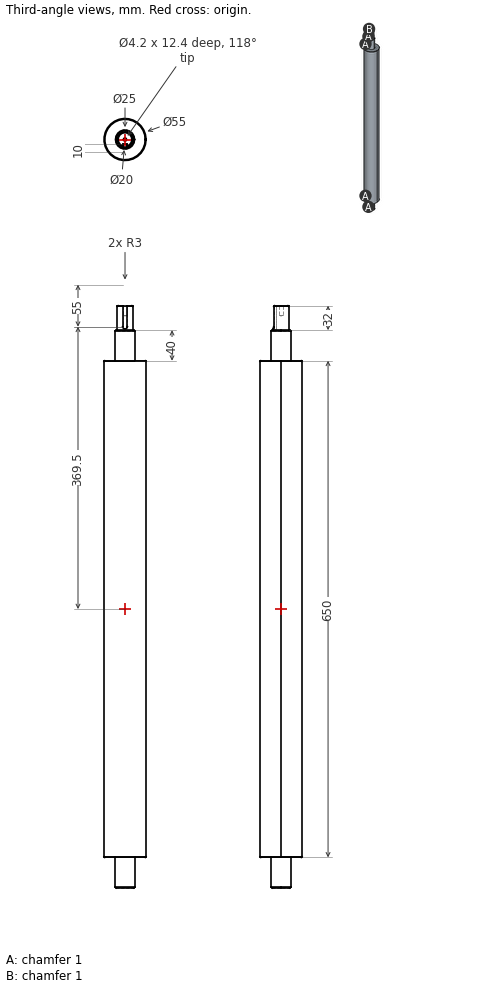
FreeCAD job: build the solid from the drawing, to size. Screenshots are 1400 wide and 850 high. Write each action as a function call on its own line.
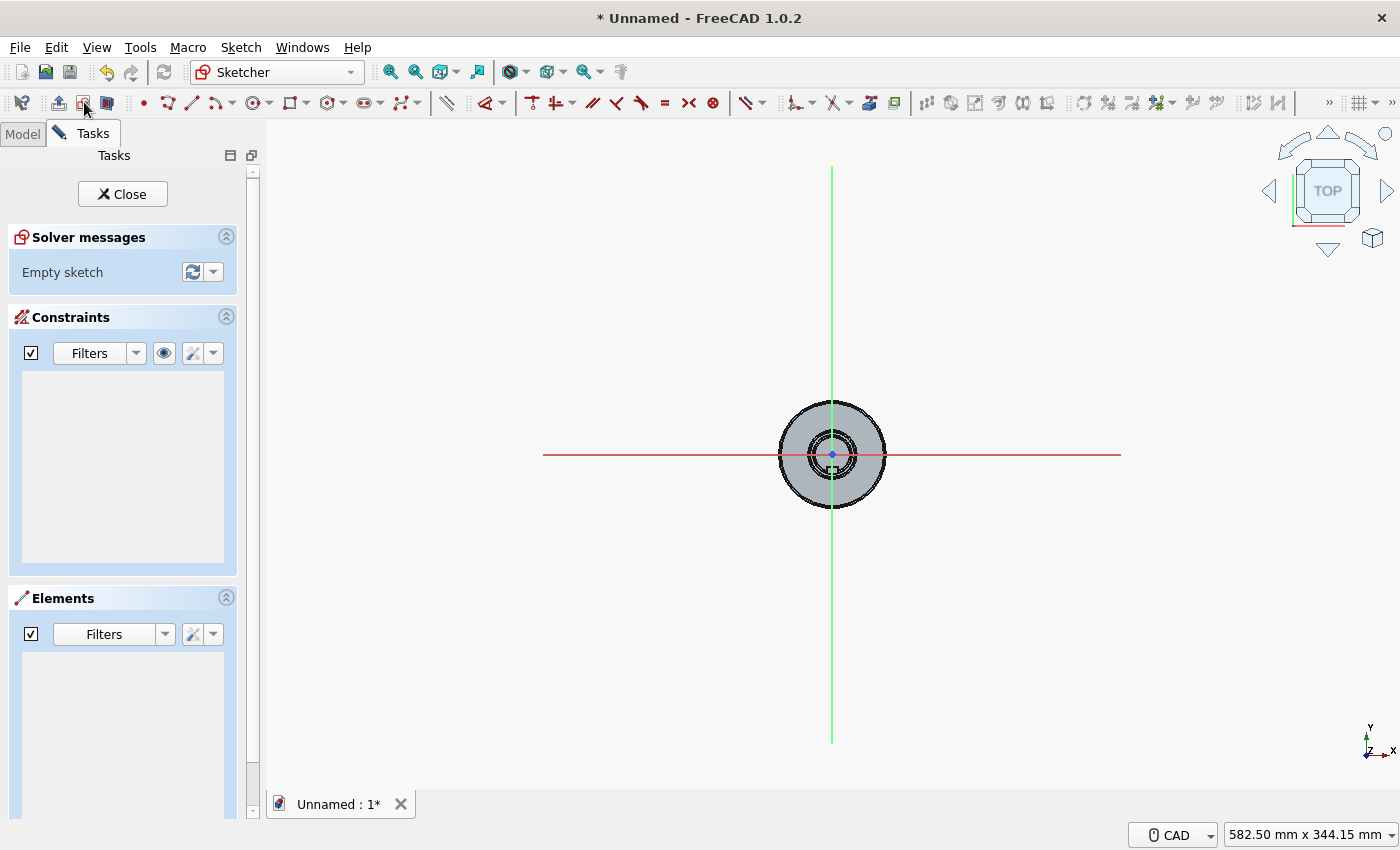
scroll(836, 455, up, 15)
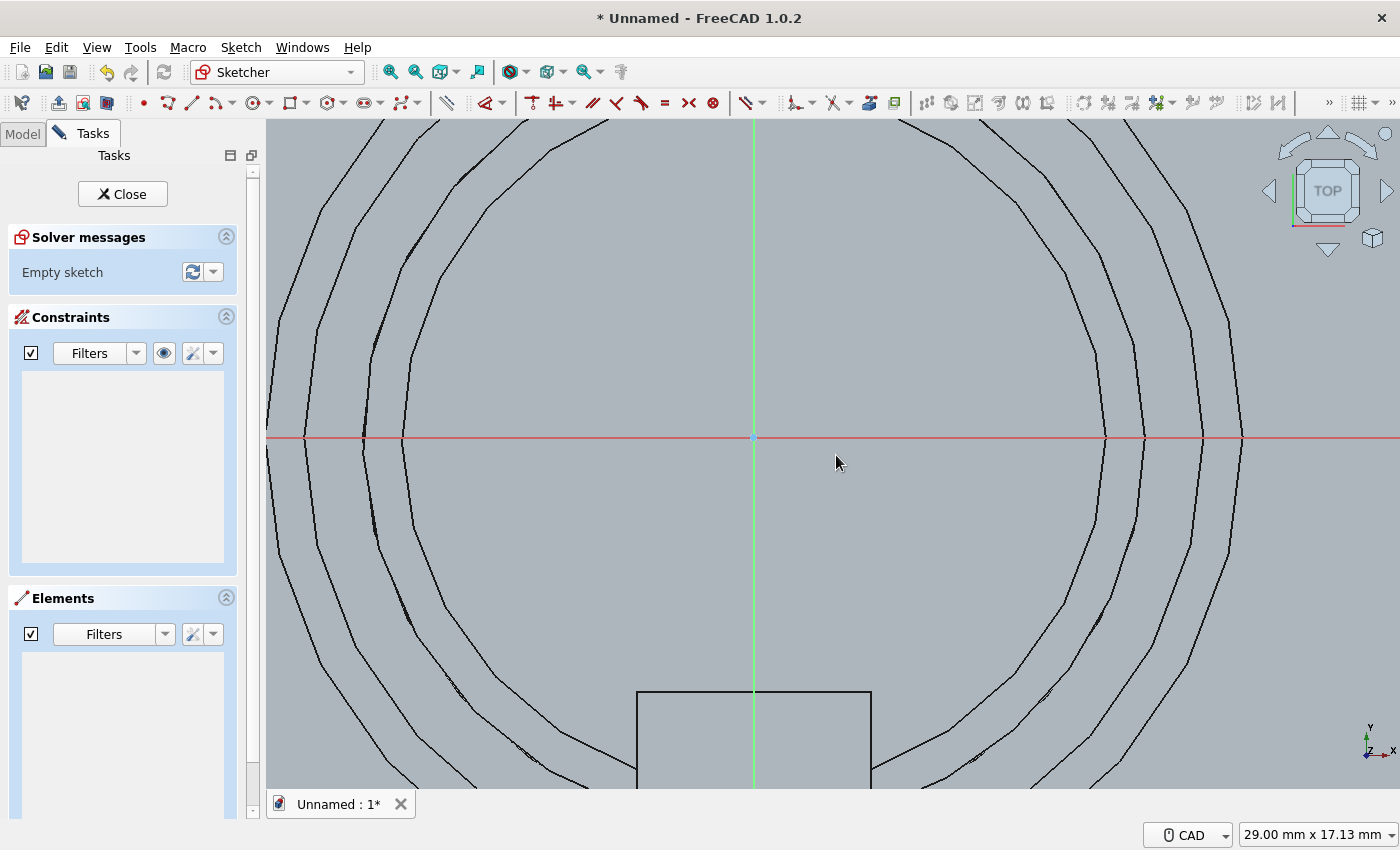
scroll(748, 428, up, 5)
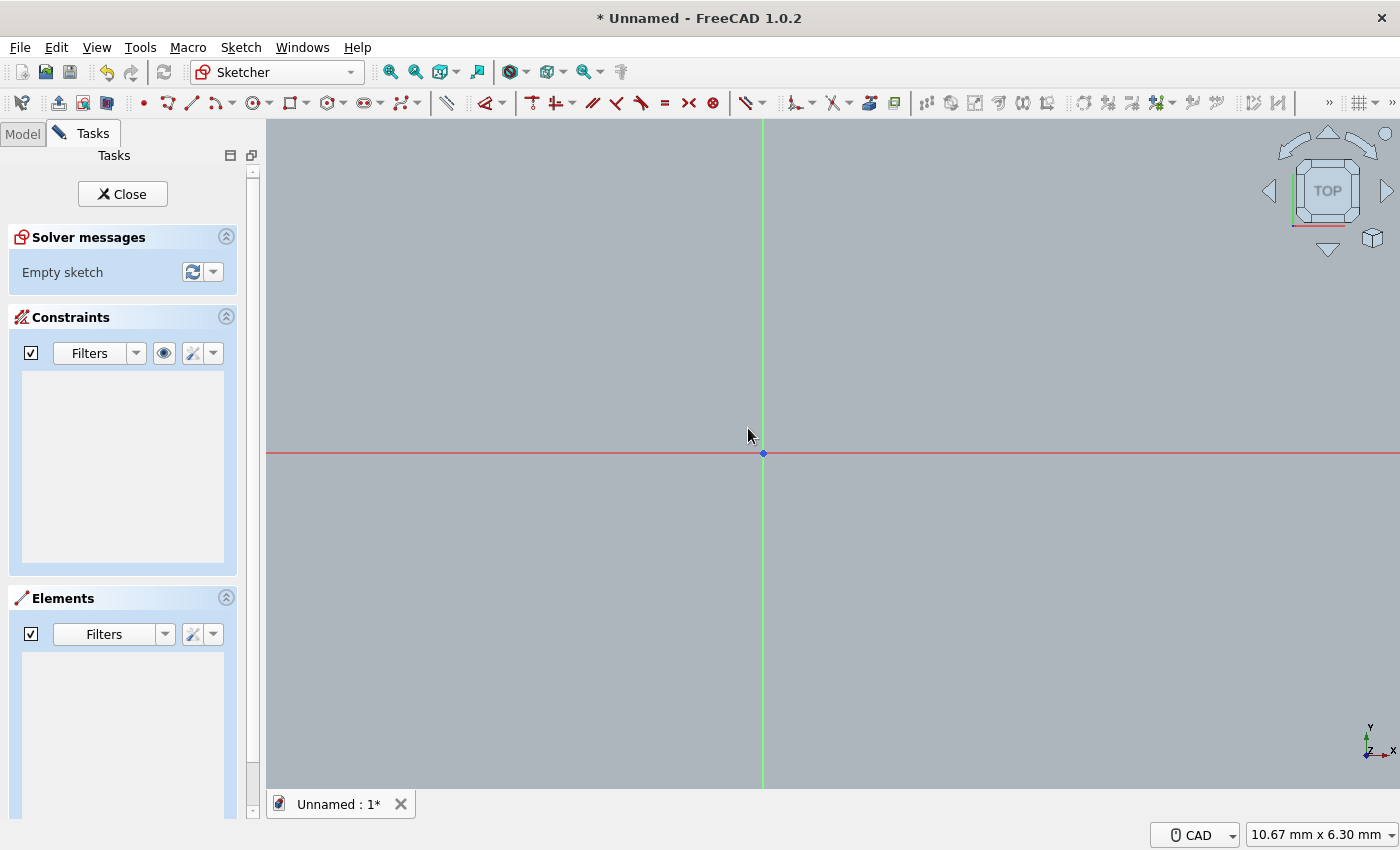
key(g)
key(c)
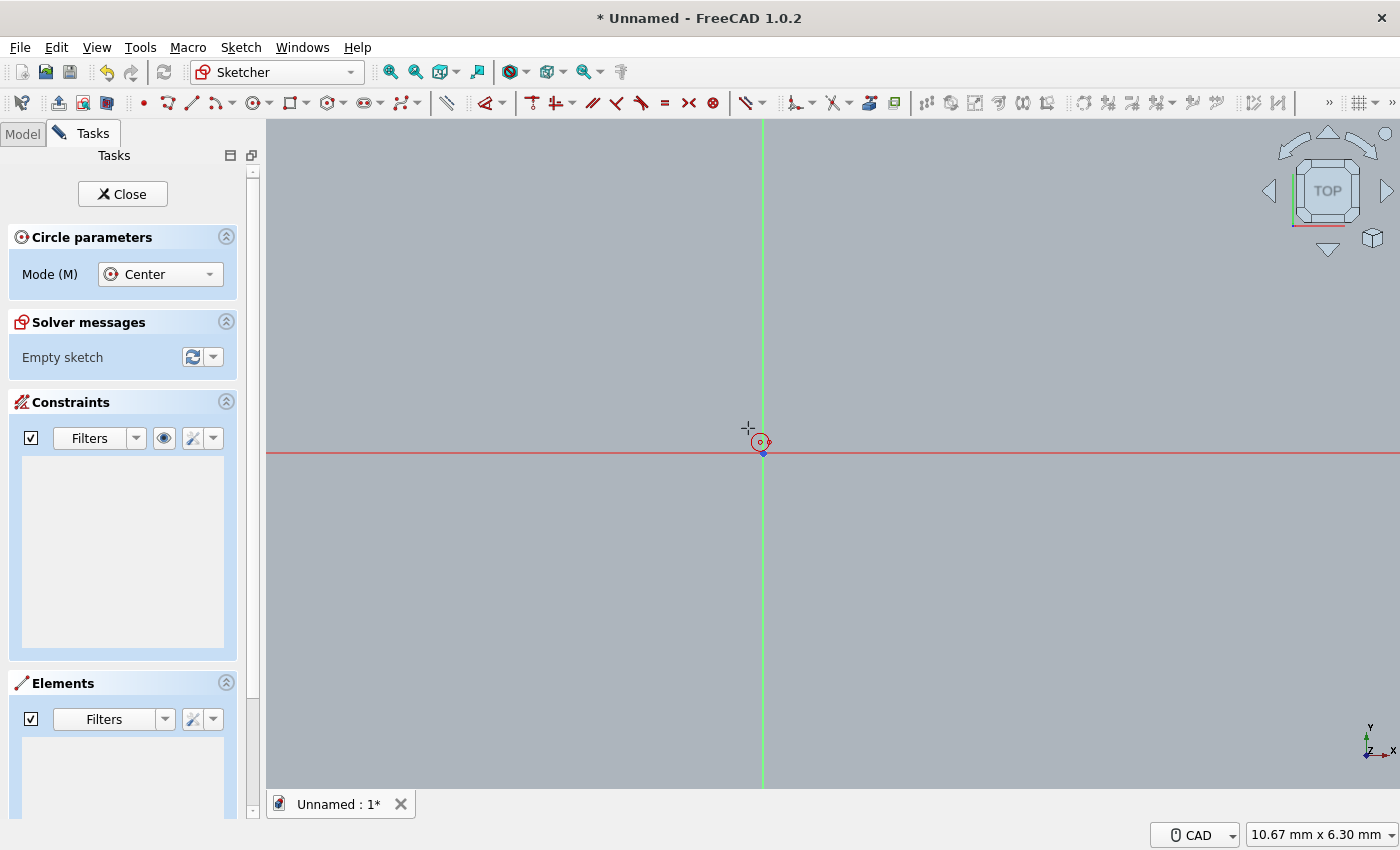
click(763, 453)
move(921, 296)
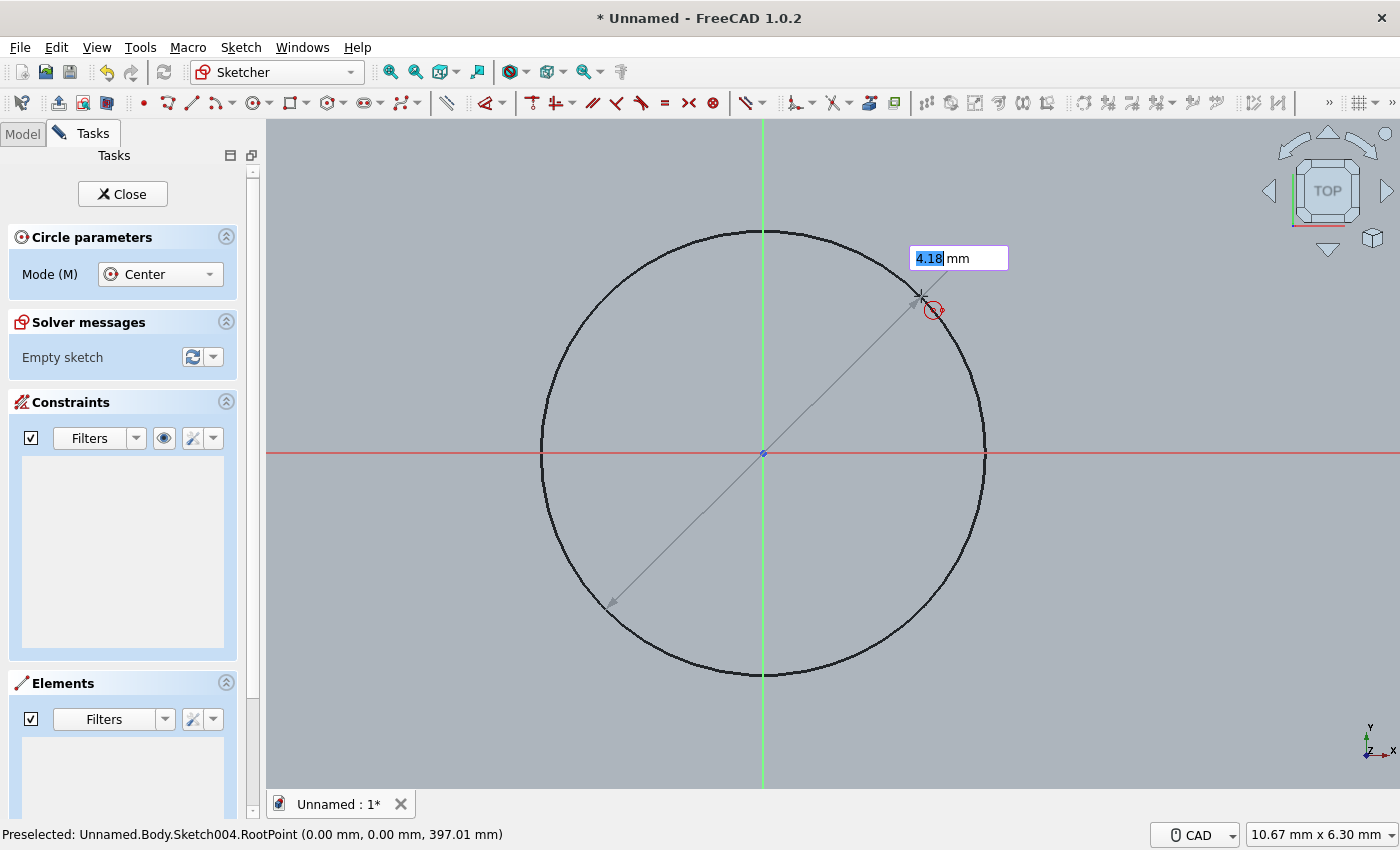
text(4.2)
key(Return)
key(Escape)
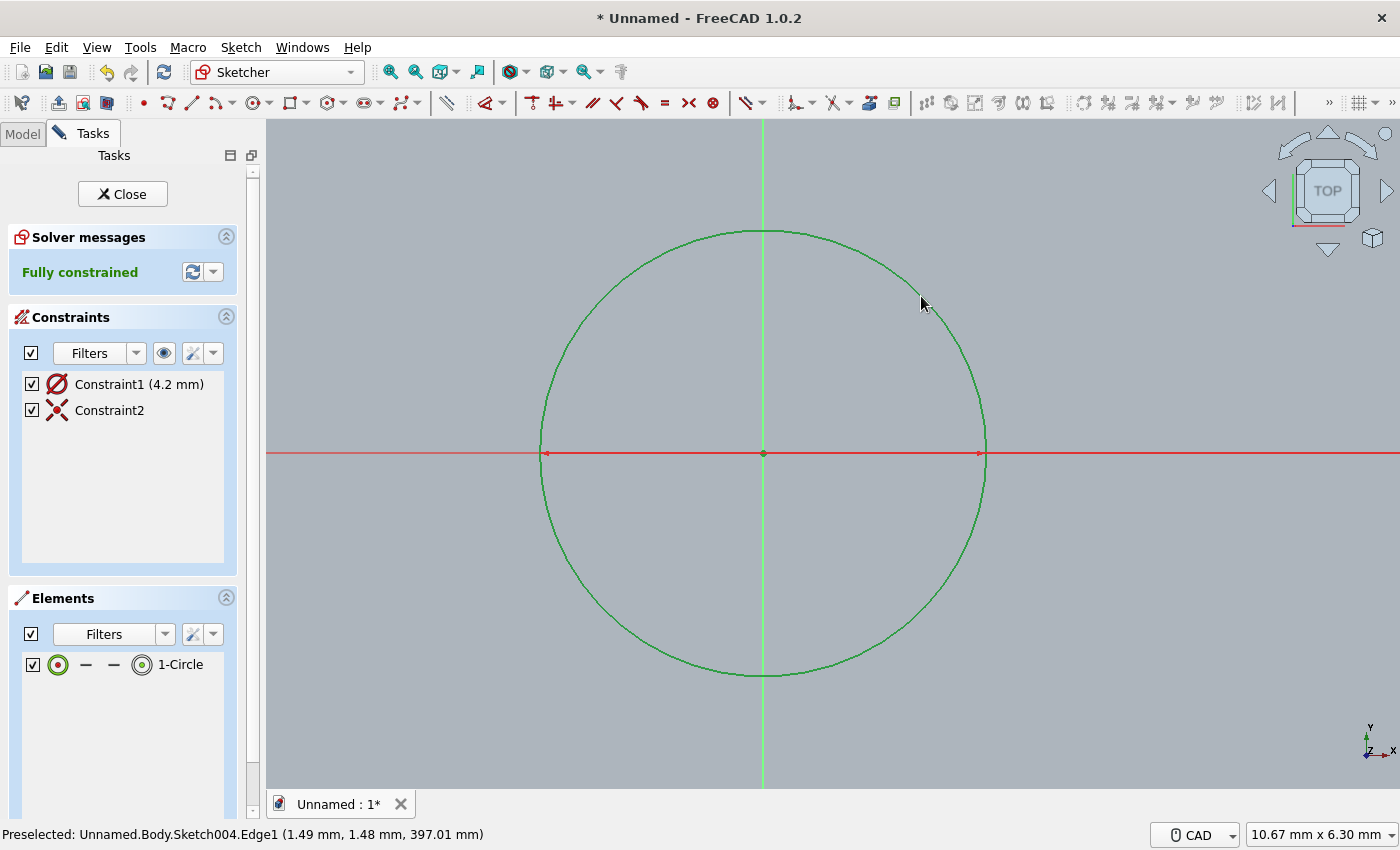
click(123, 194)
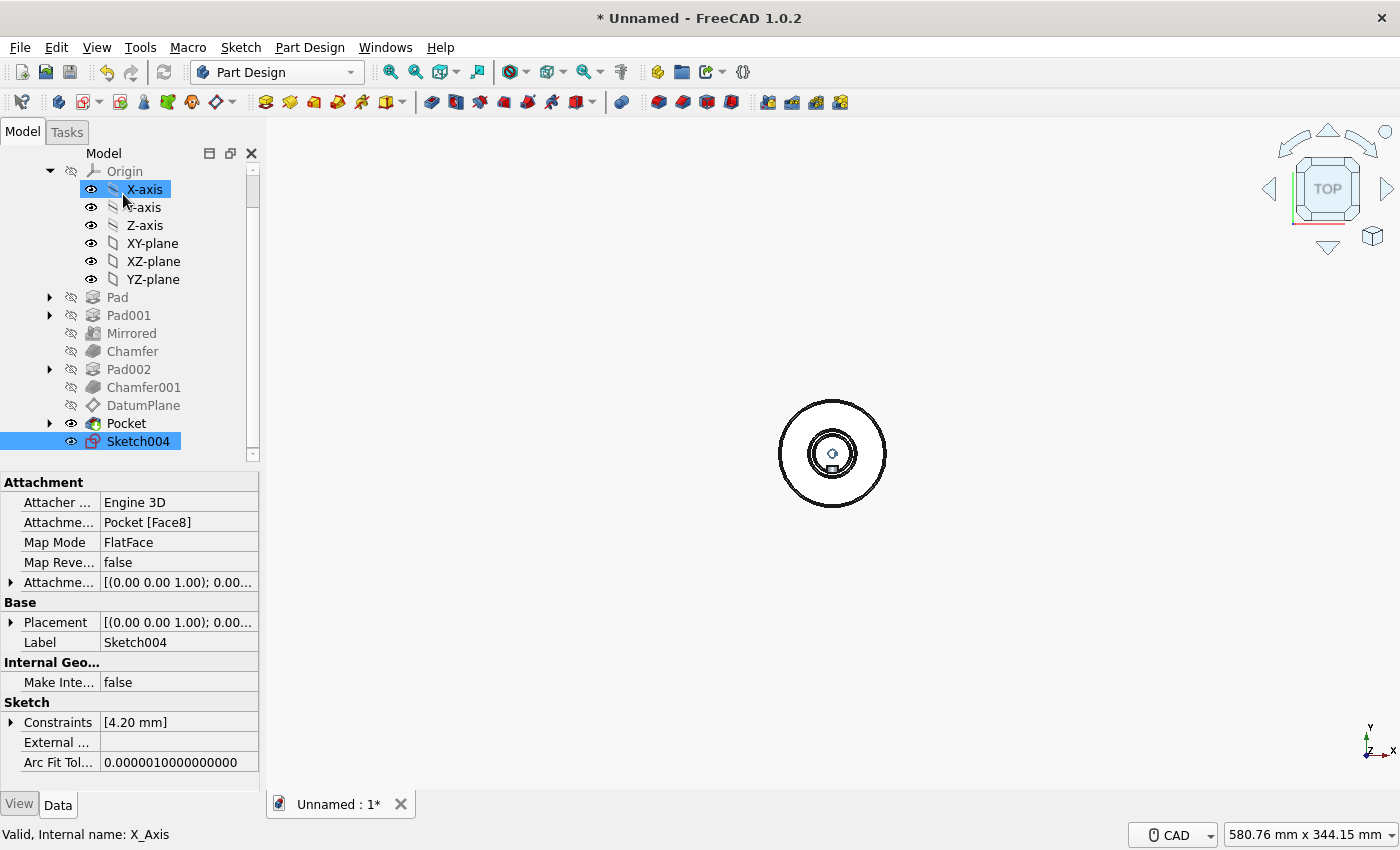
click(456, 102)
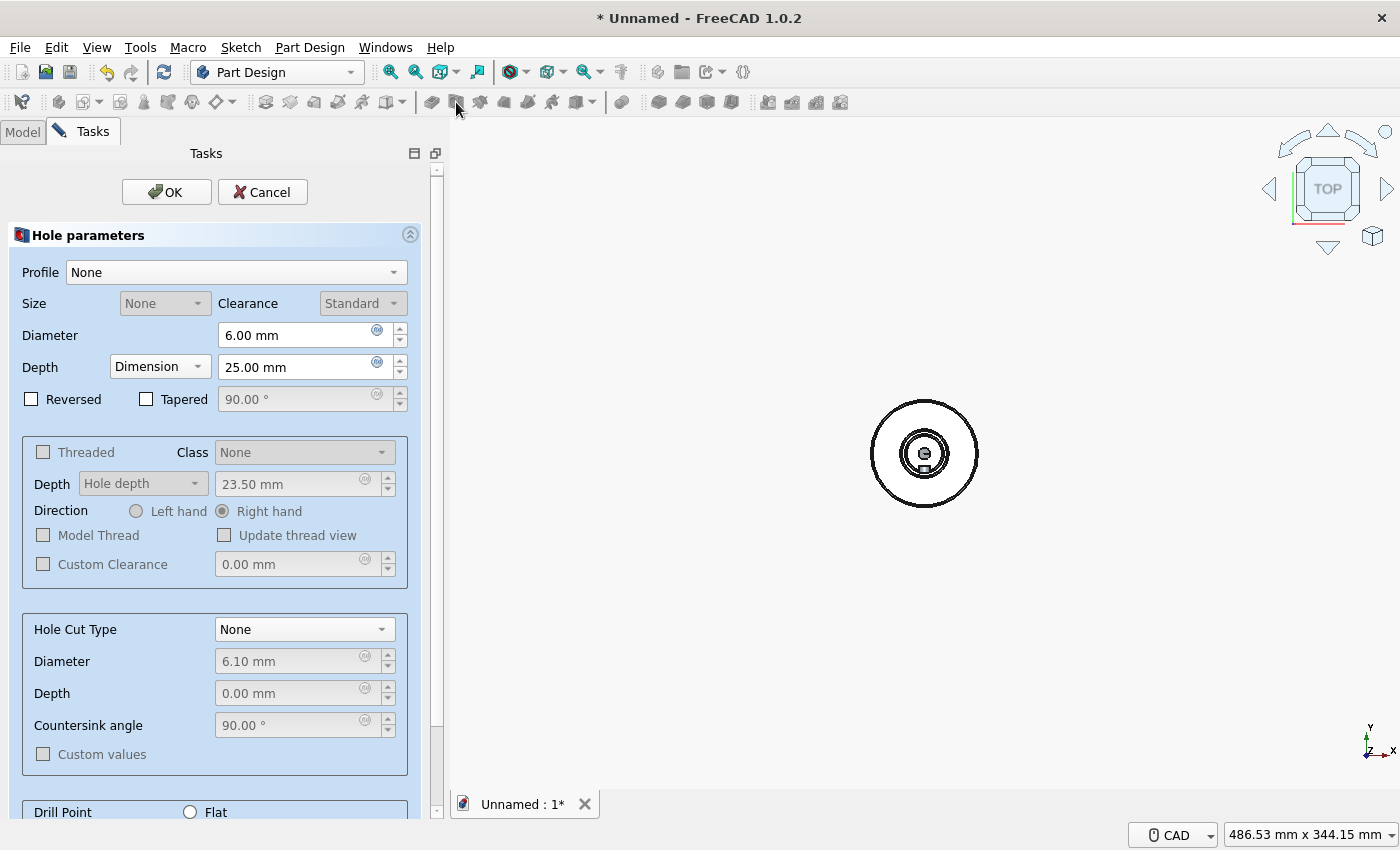
triple_click(305, 335)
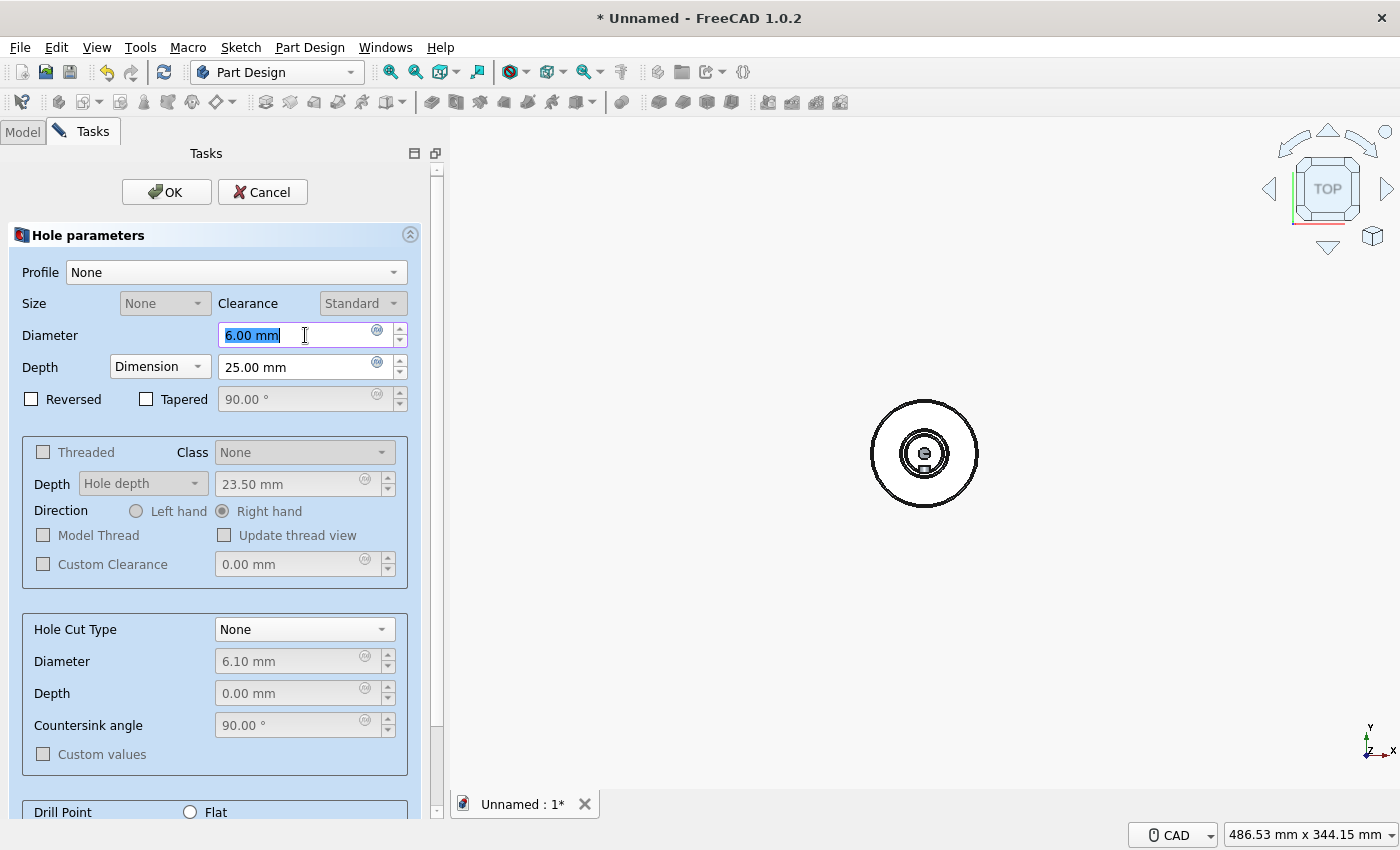
text(4.2)
key(Tab)